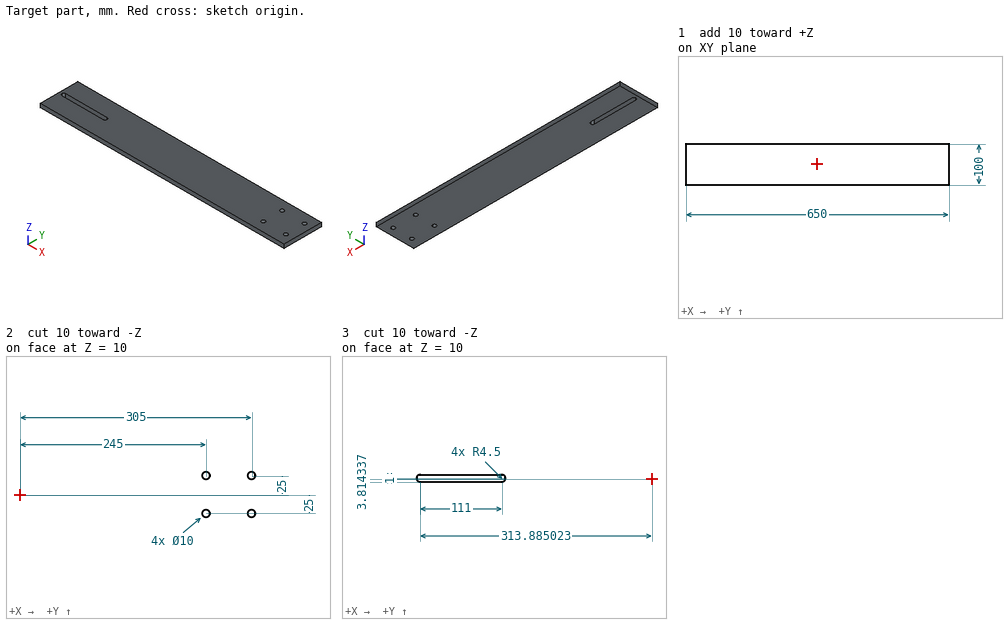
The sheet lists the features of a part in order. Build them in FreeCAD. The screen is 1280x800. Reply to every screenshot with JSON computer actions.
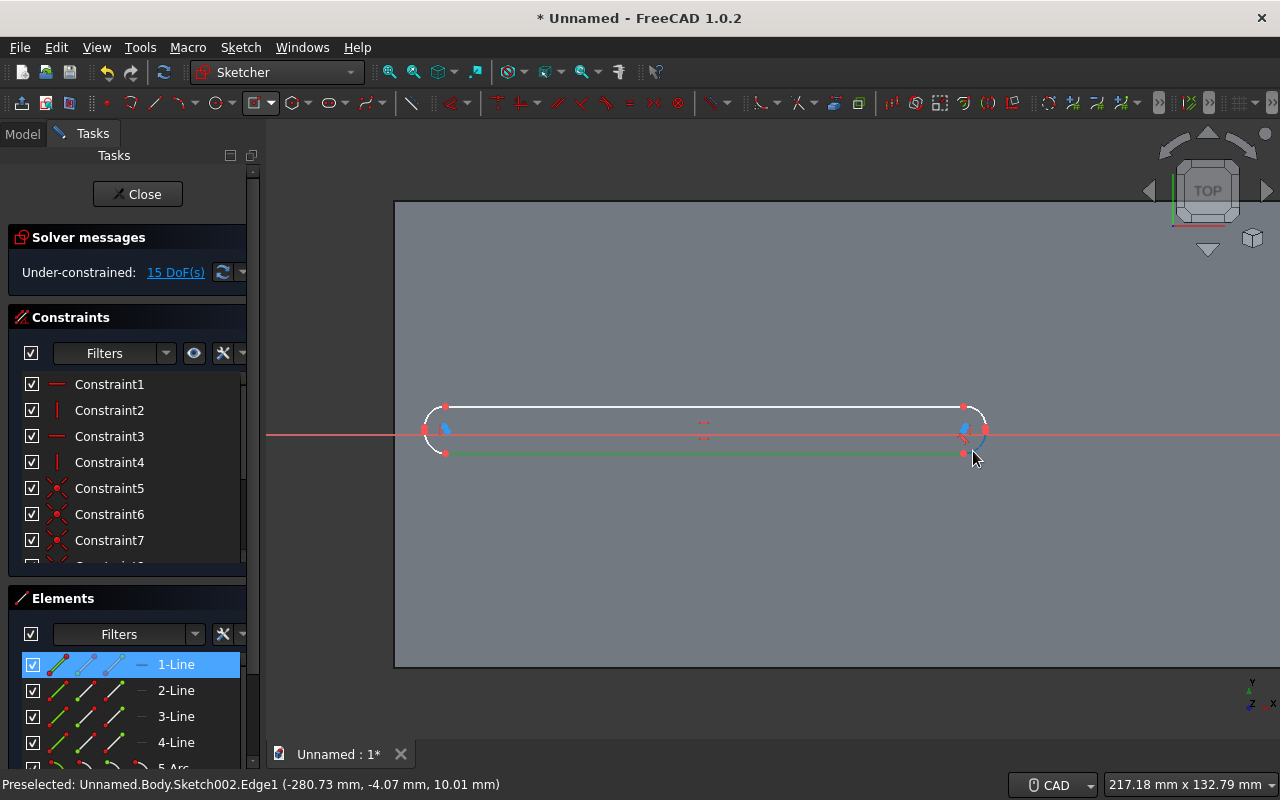
{"action": "scroll", "coordinate": [427, 441], "scroll_direction": "up", "scroll_amount": 4}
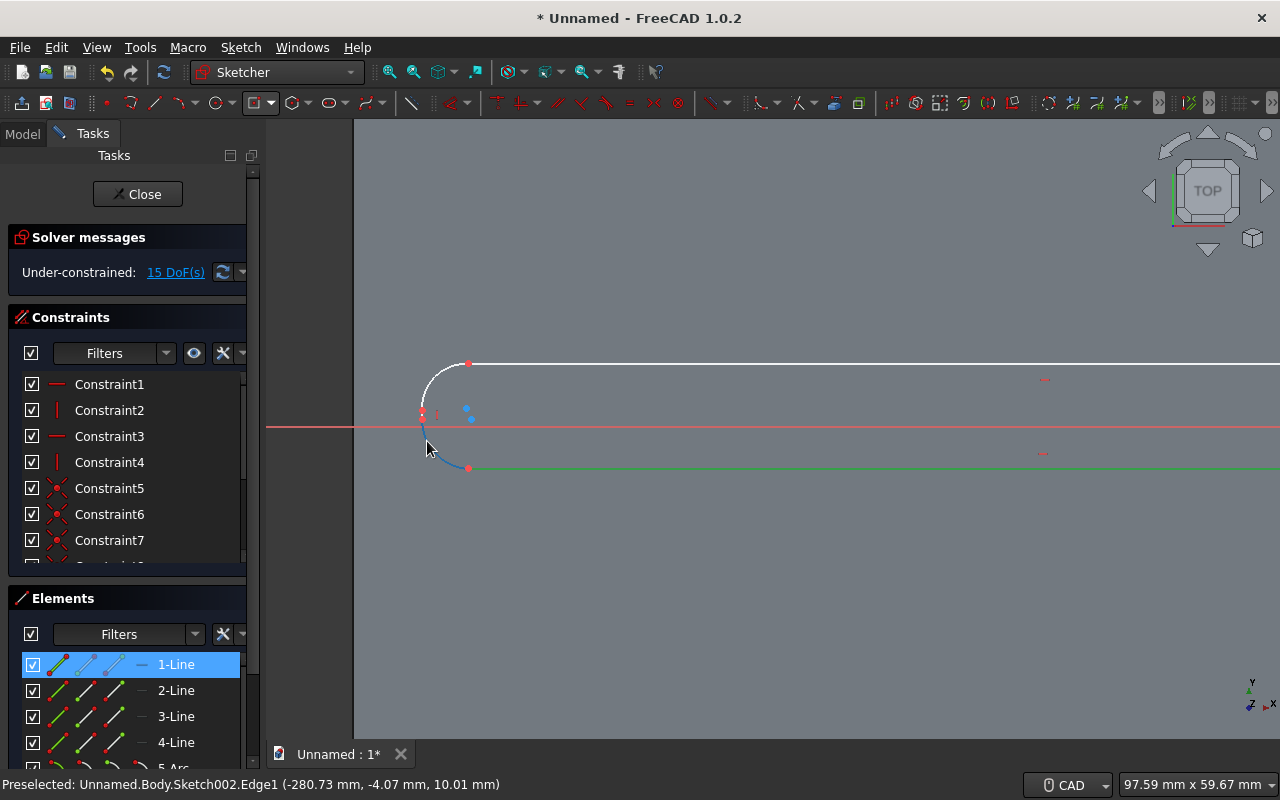
{"action": "left_click", "coordinate": [427, 441]}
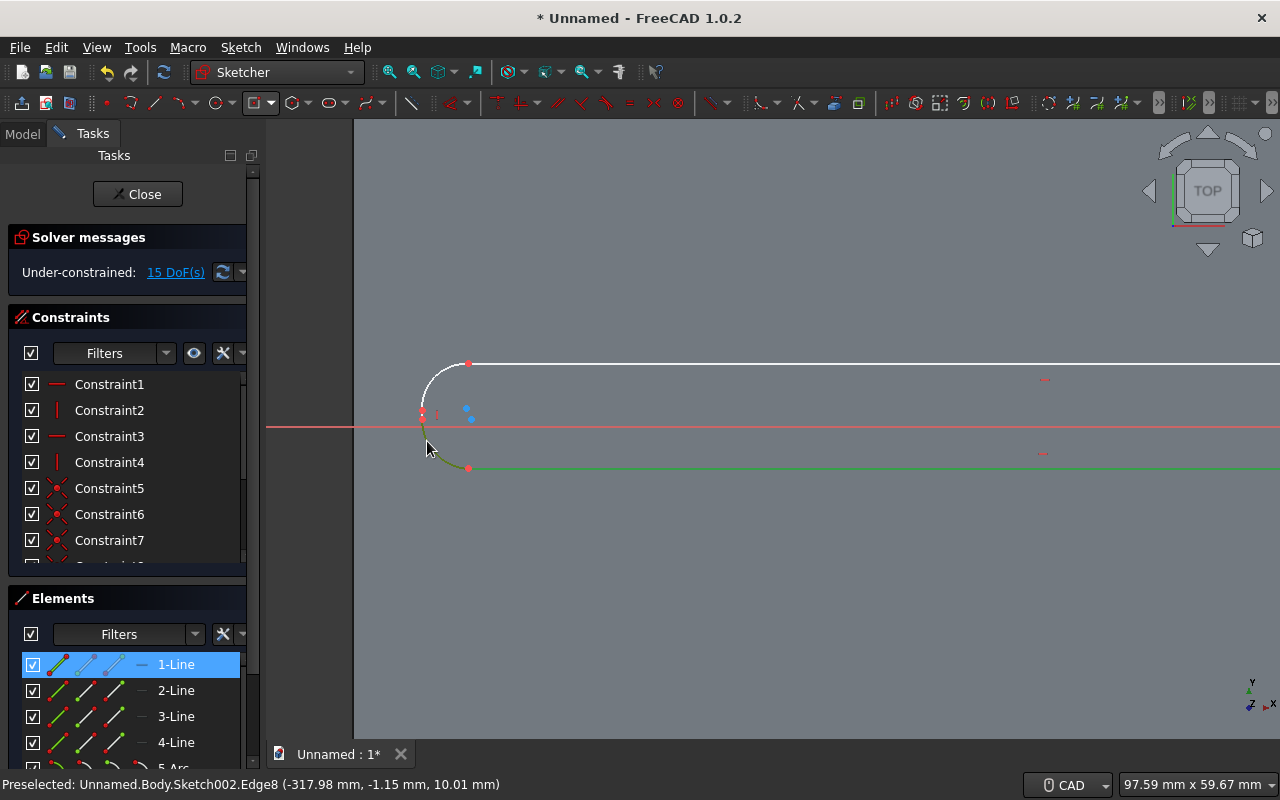
{"action": "left_click", "coordinate": [606, 104]}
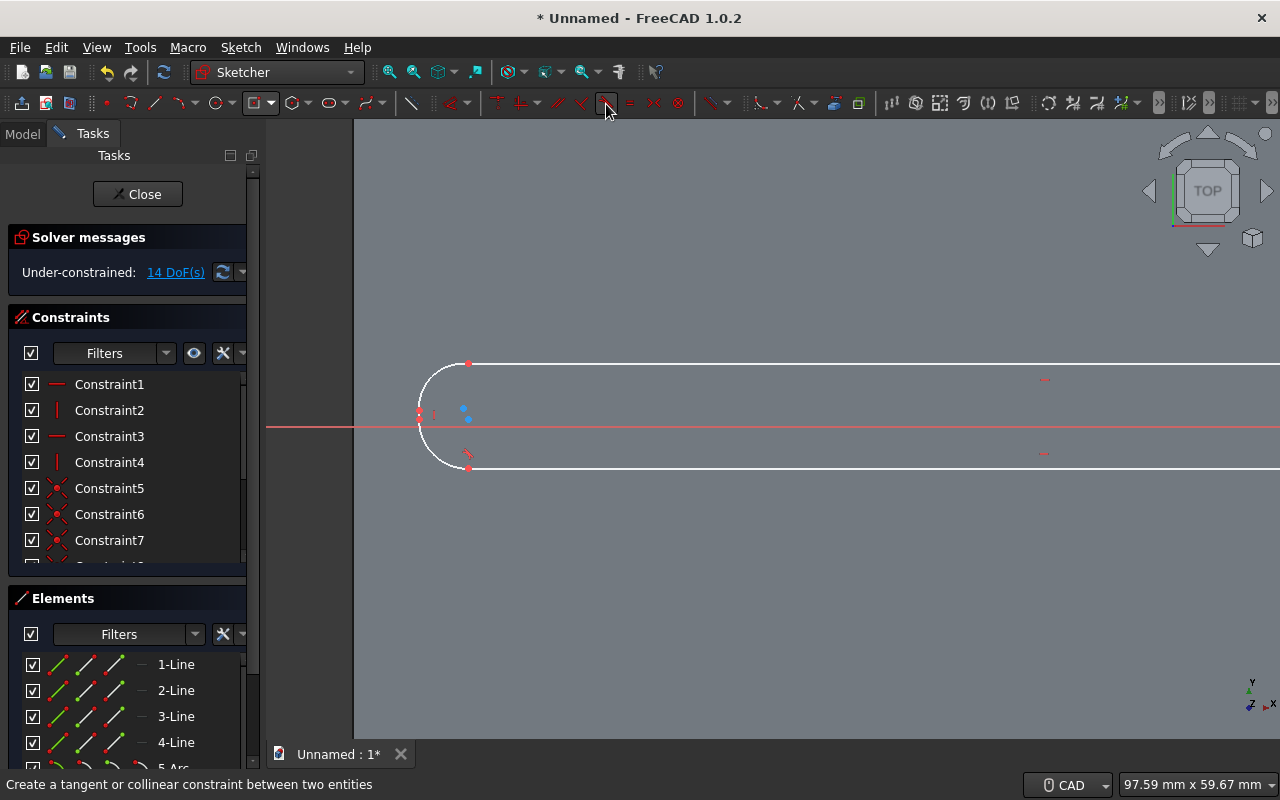
{"action": "scroll", "coordinate": [426, 441], "scroll_direction": "down", "scroll_amount": 4}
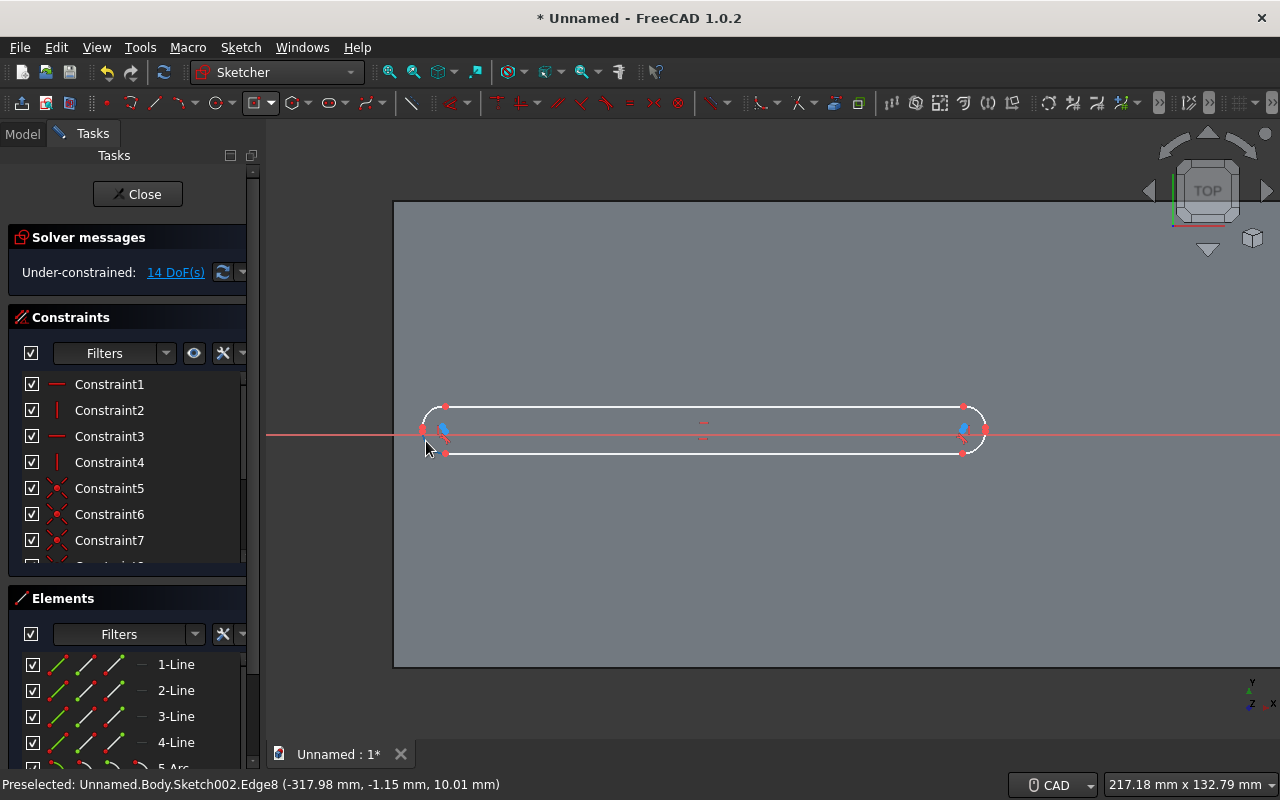
{"action": "scroll", "coordinate": [985, 429], "scroll_direction": "up", "scroll_amount": 9}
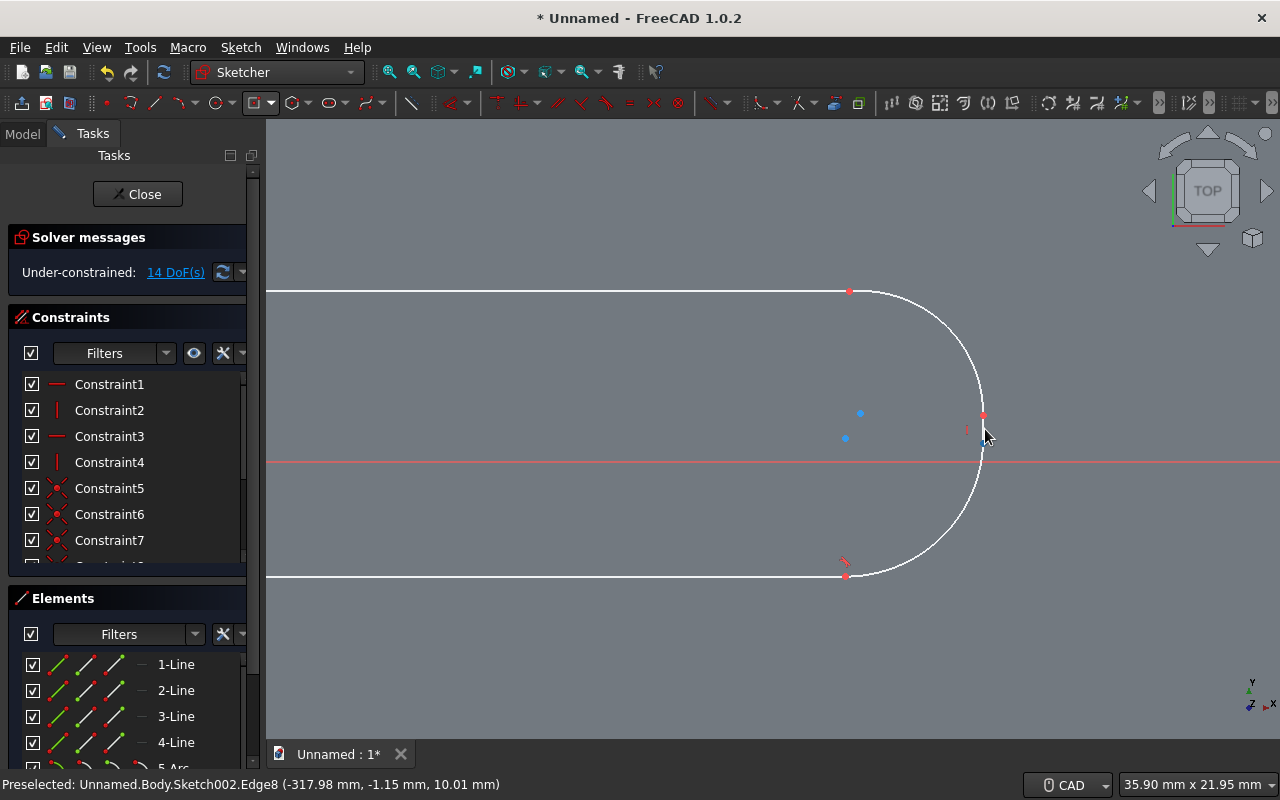
{"action": "left_click", "coordinate": [983, 429]}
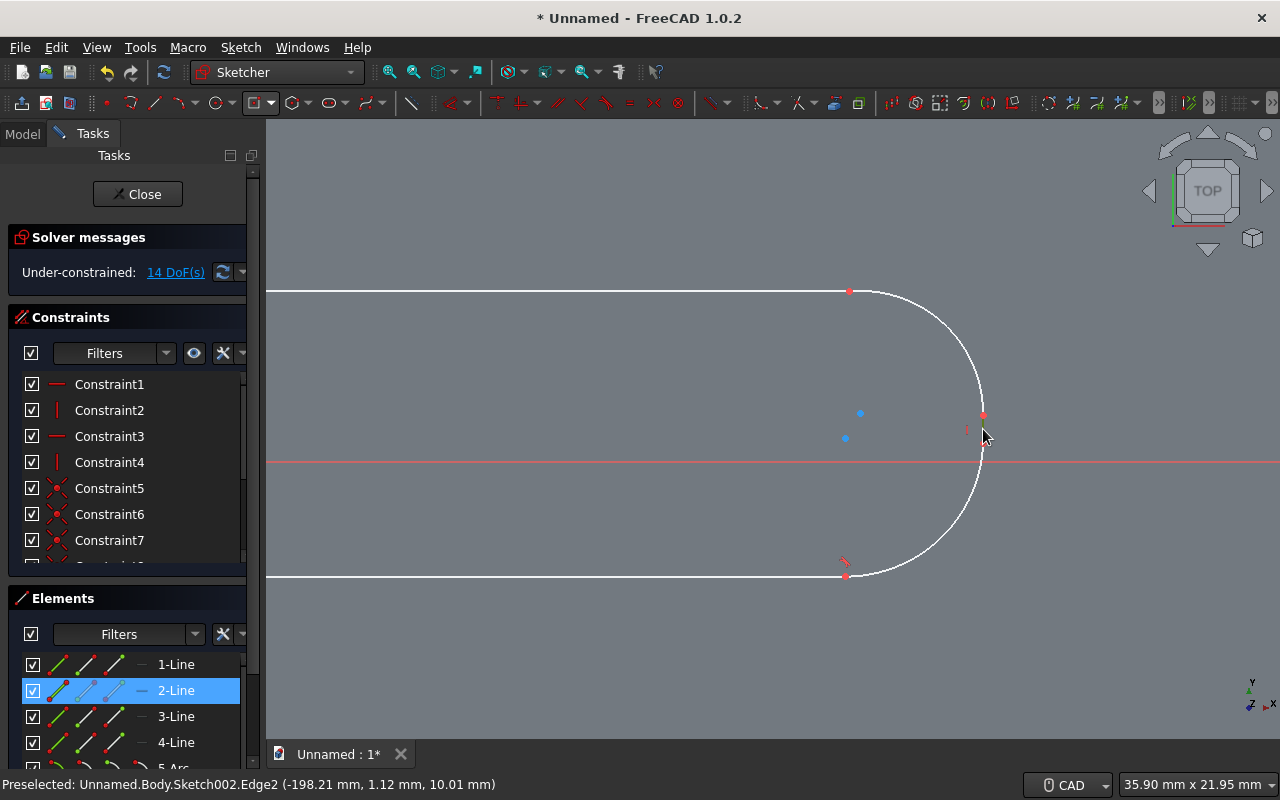
{"action": "scroll", "coordinate": [986, 429], "scroll_direction": "down", "scroll_amount": 9}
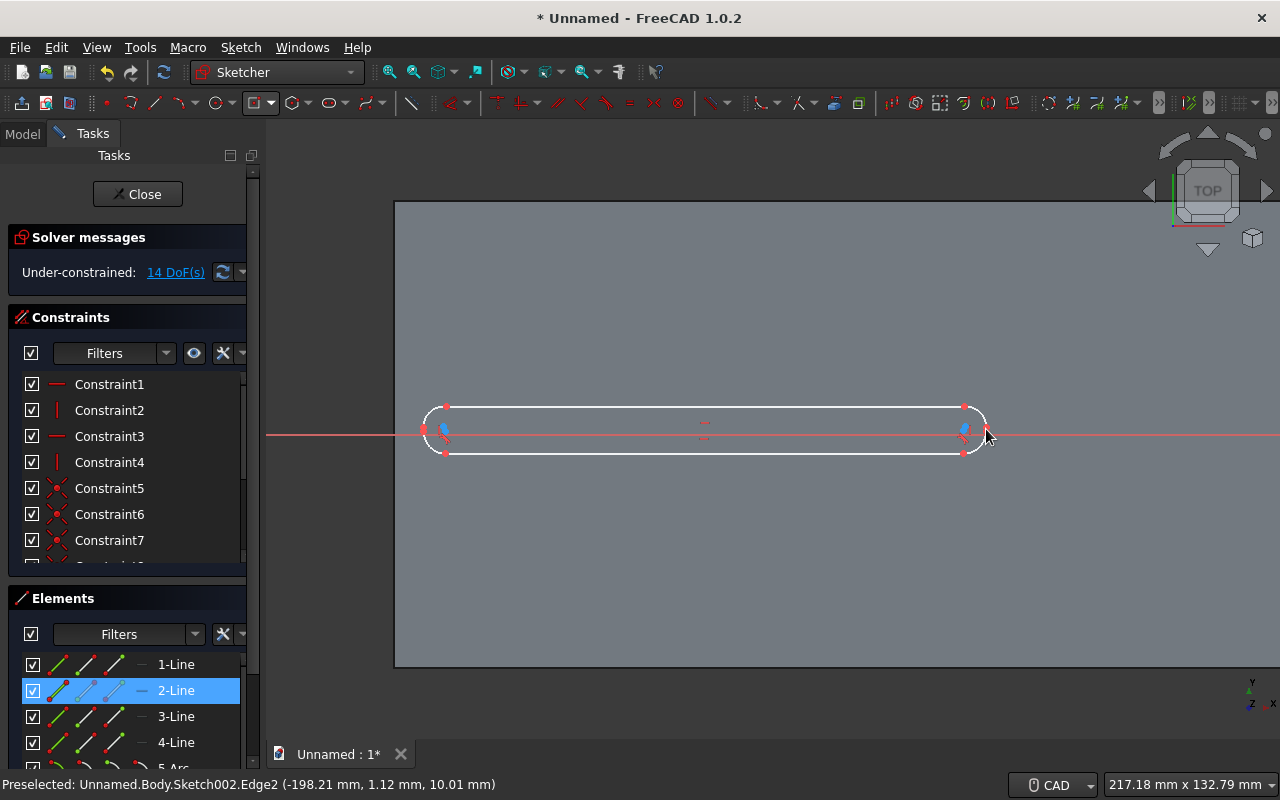
{"action": "scroll", "coordinate": [973, 451], "scroll_direction": "up", "scroll_amount": 2}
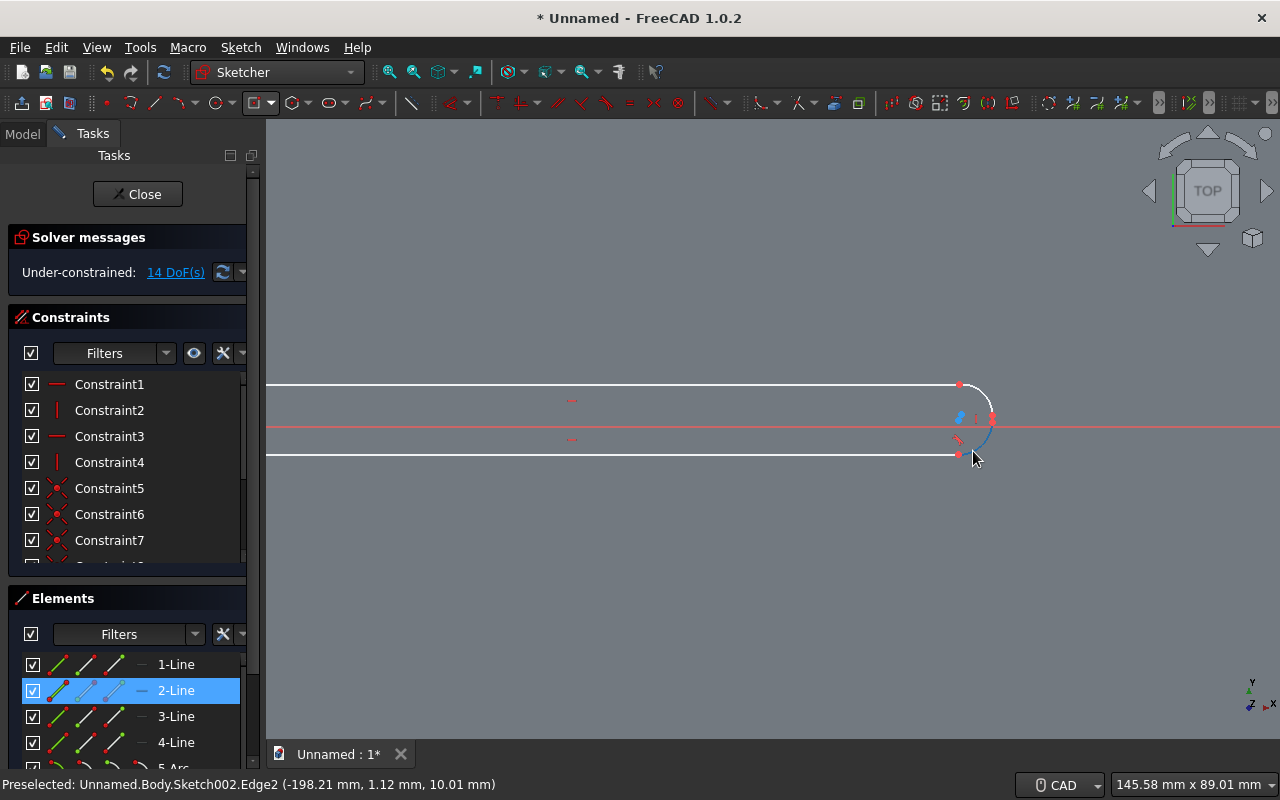
{"action": "left_click", "coordinate": [973, 451]}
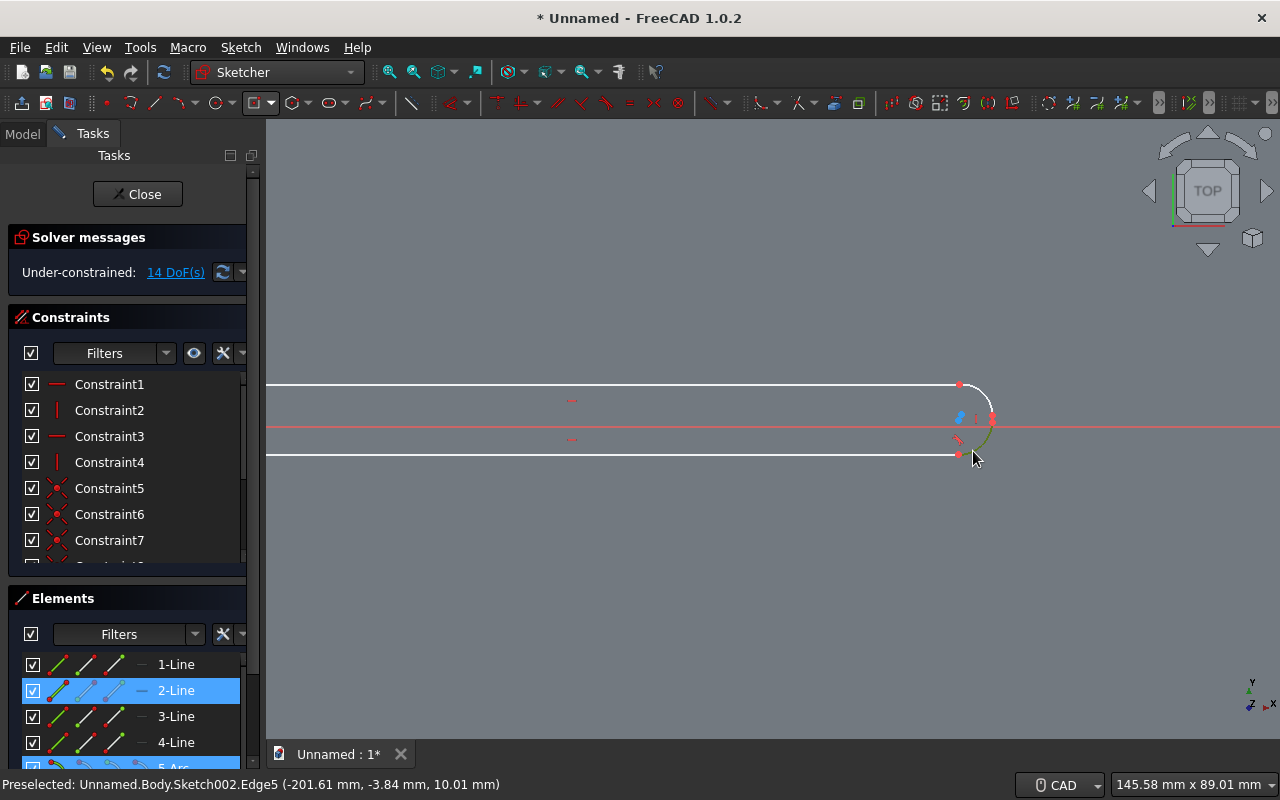
{"action": "key", "text": "t"}